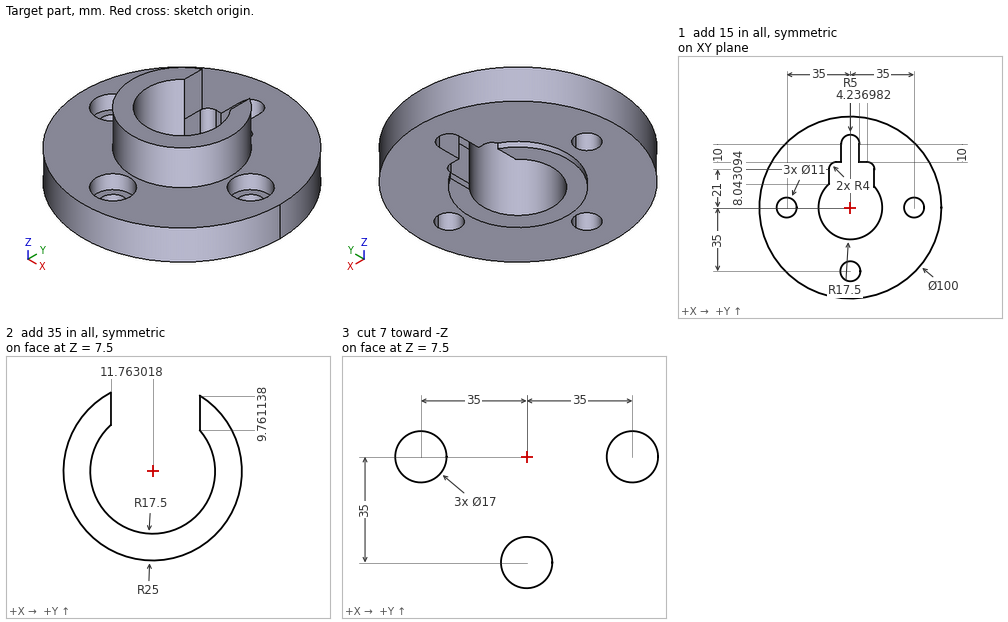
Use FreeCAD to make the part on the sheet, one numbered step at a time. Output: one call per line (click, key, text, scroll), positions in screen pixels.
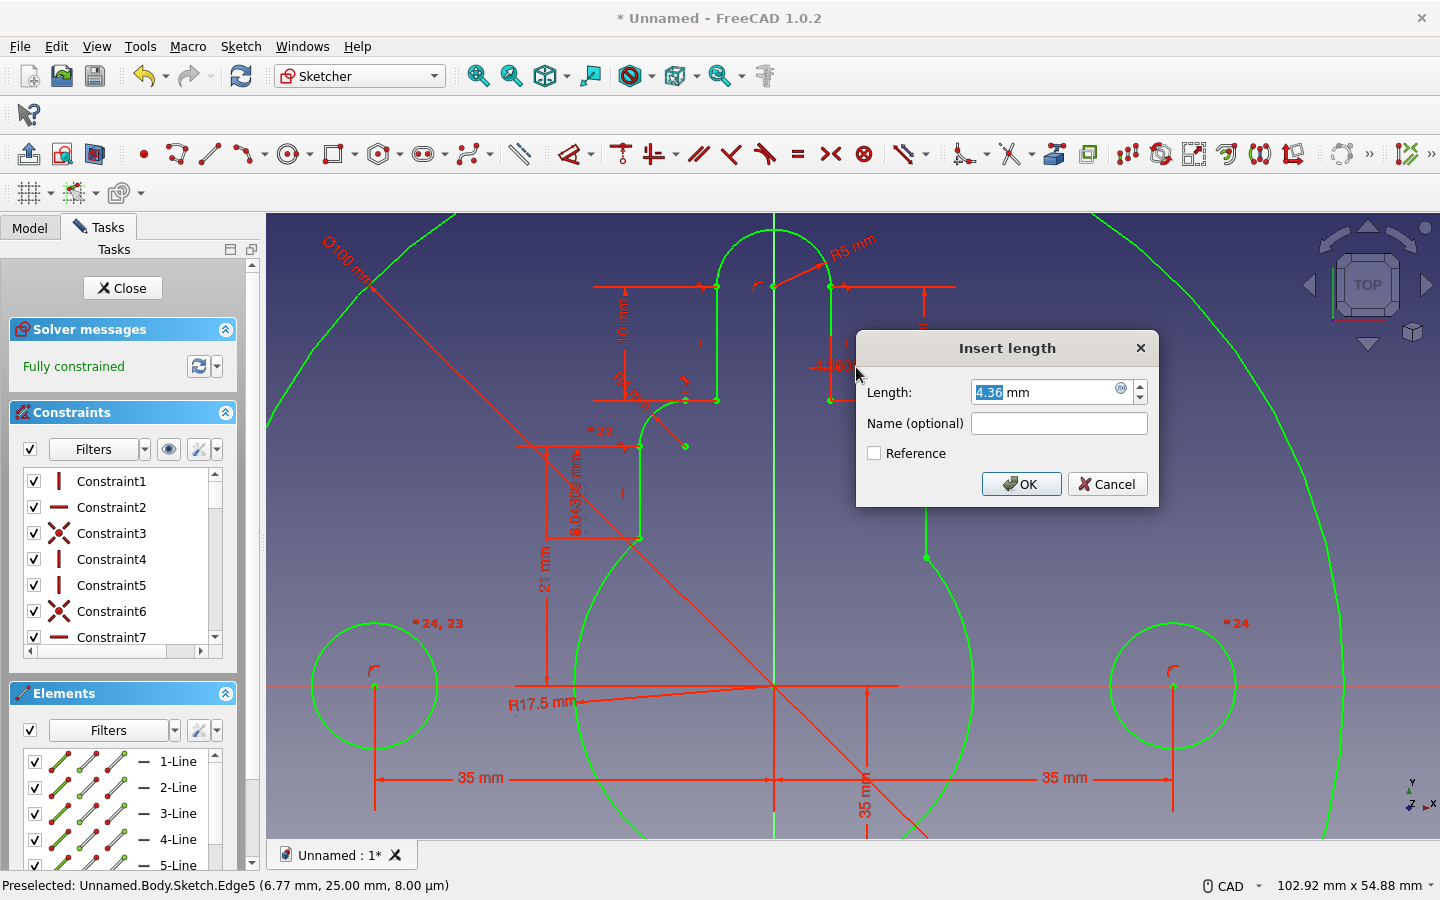
text(4.236982)
key(Return)
key(Escape)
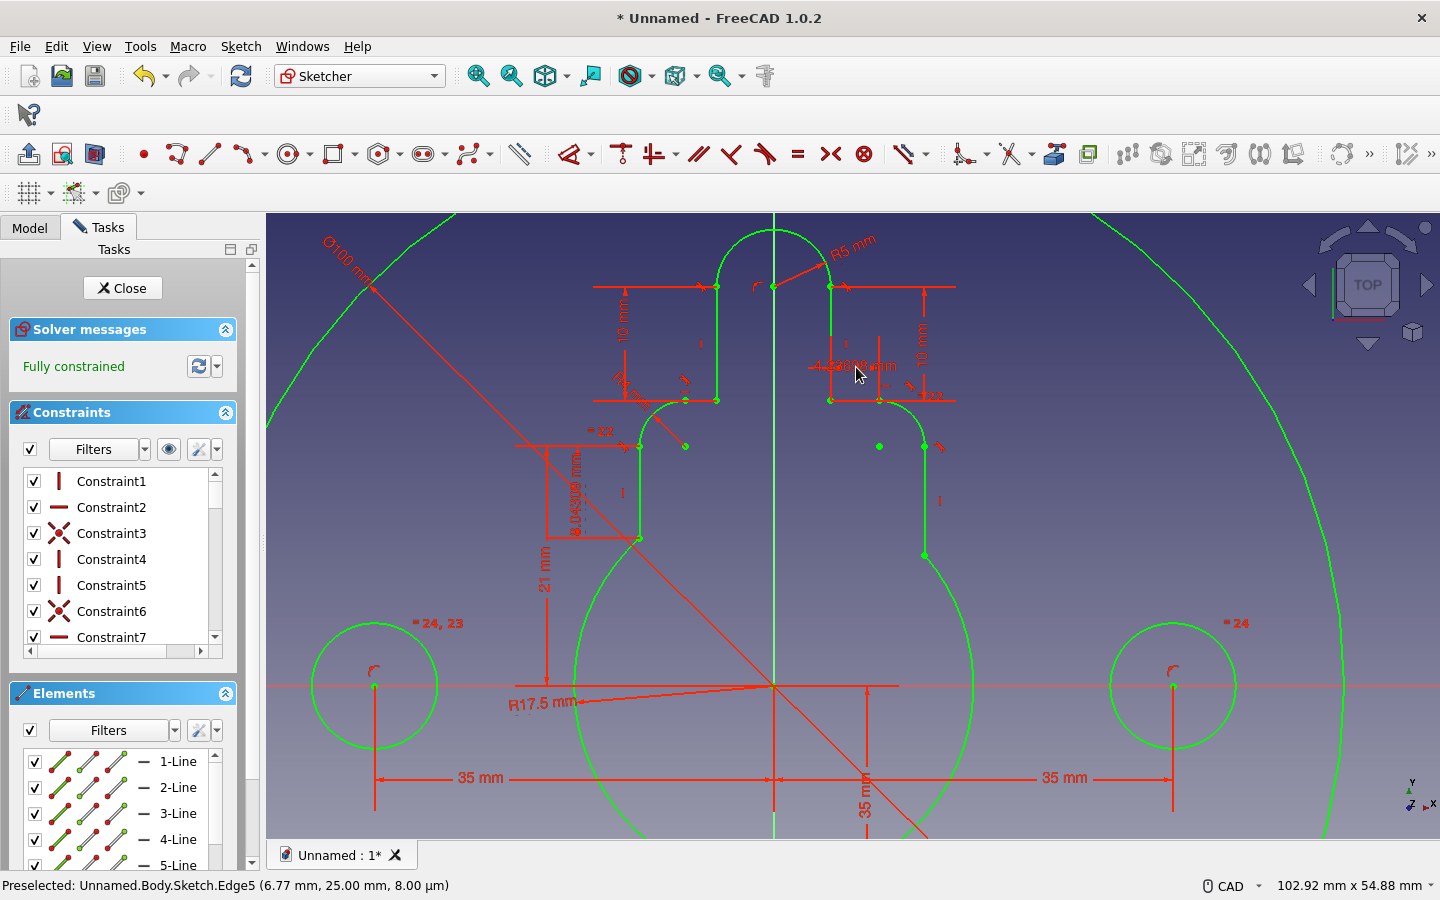
click(123, 288)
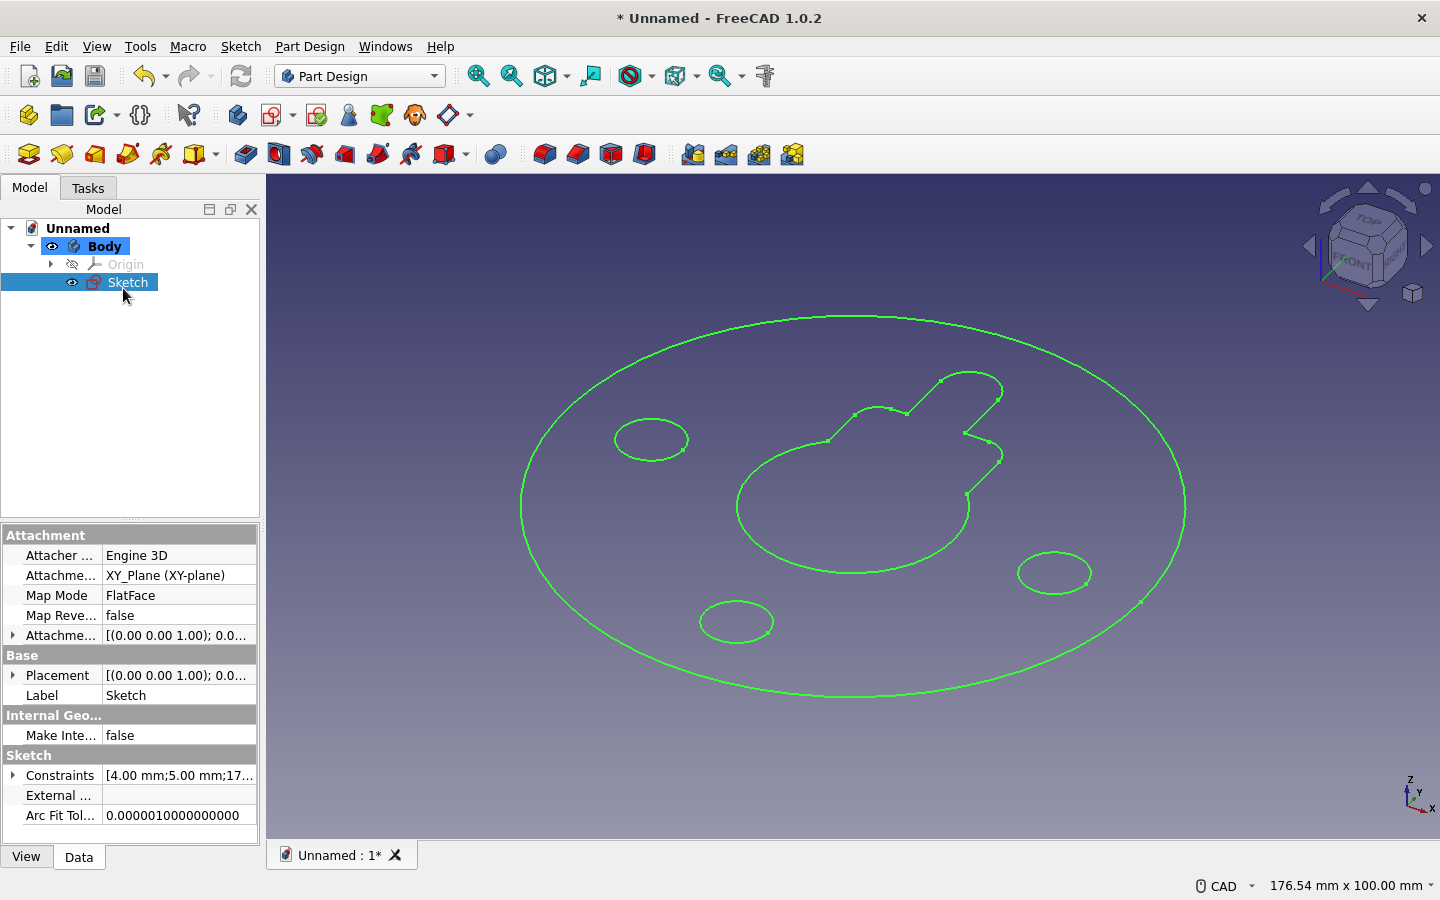
click(29, 154)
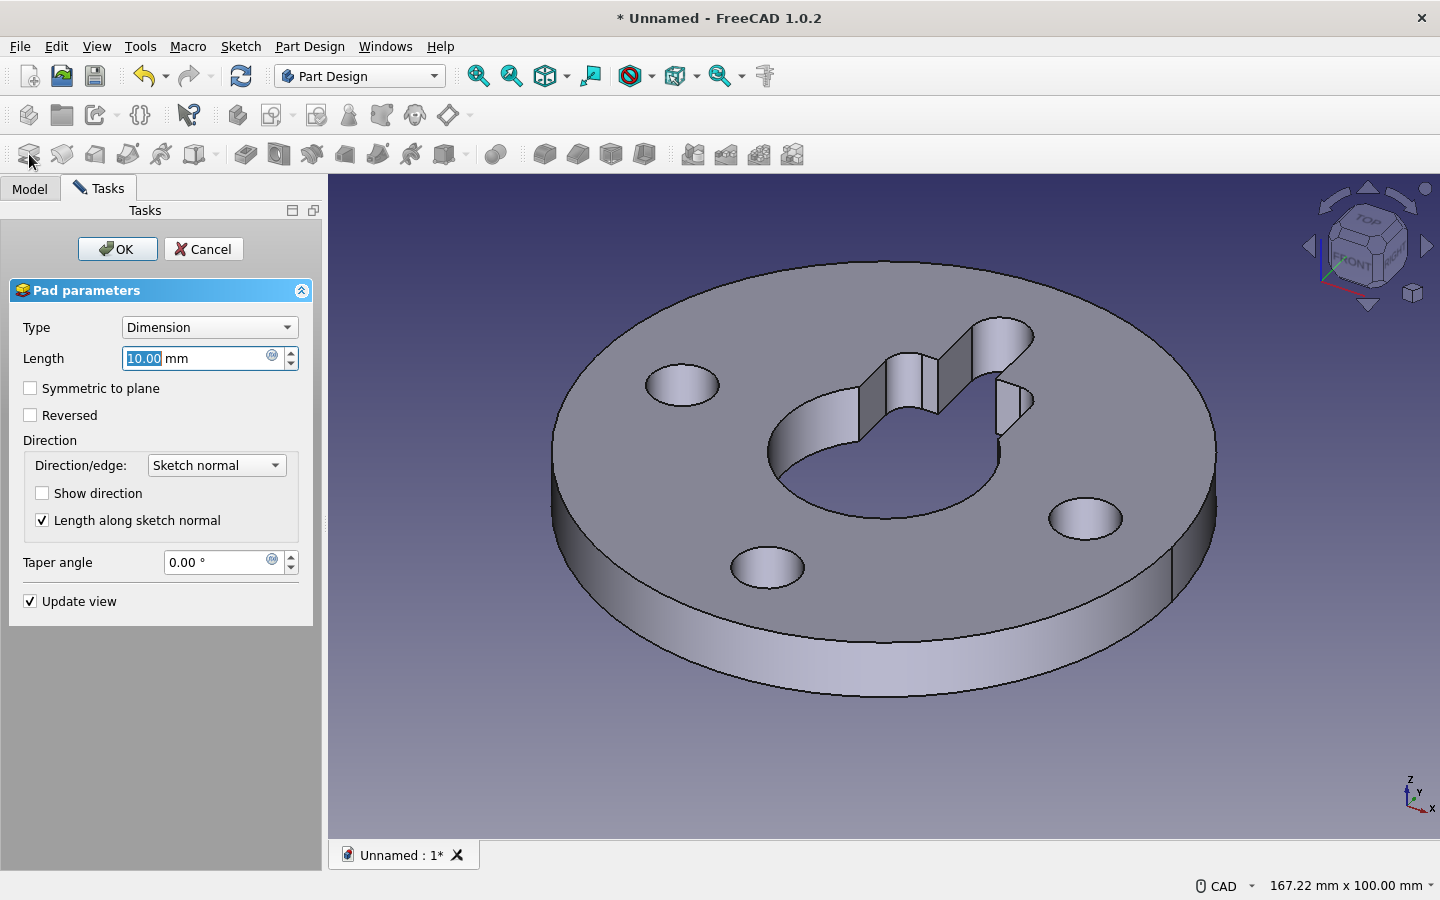
text(15)
key(Tab)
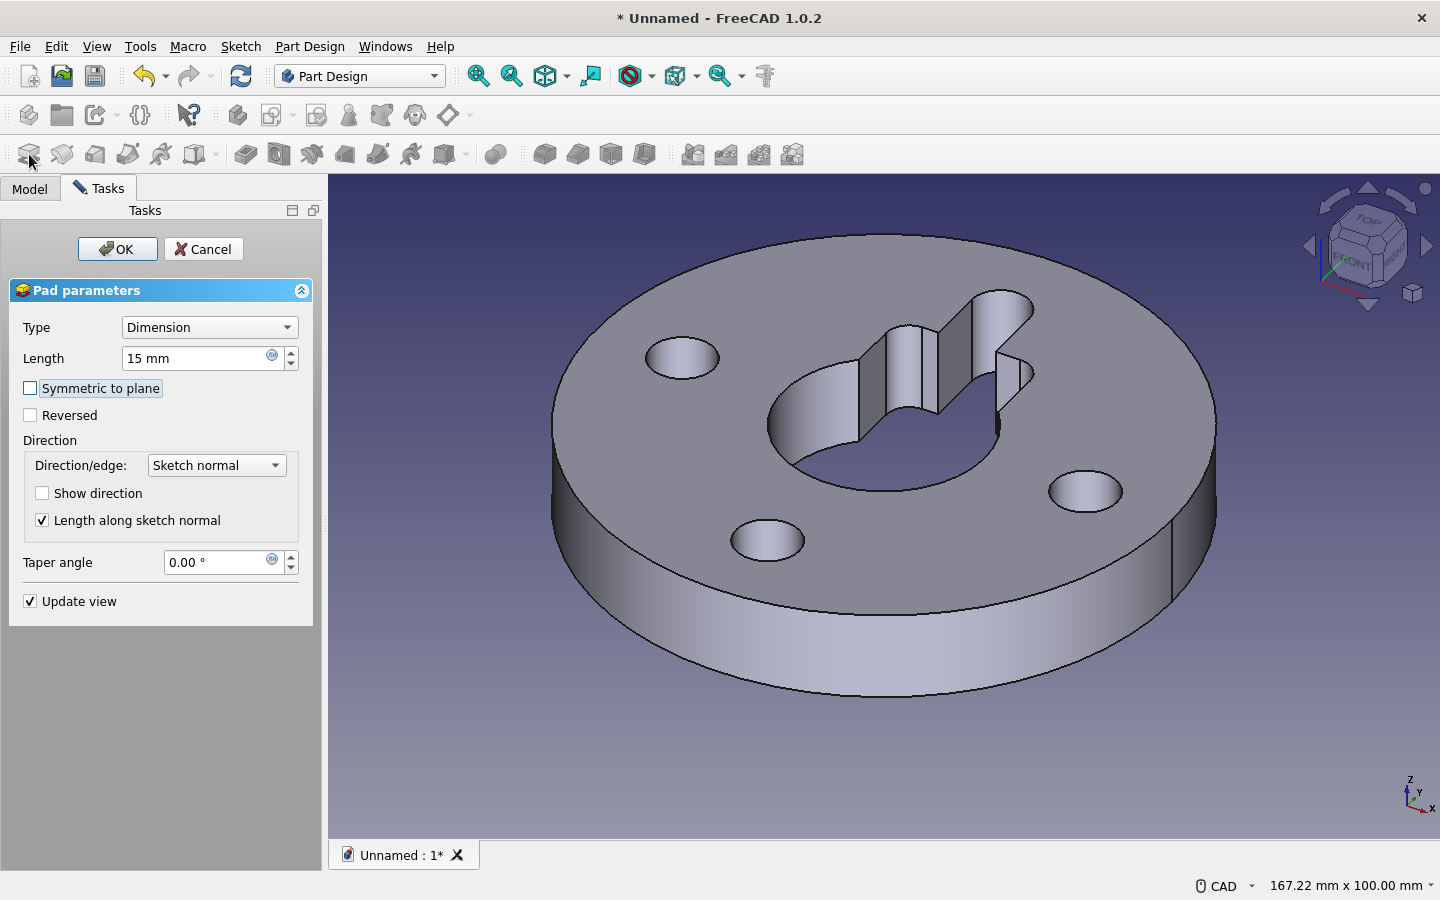
click(31, 388)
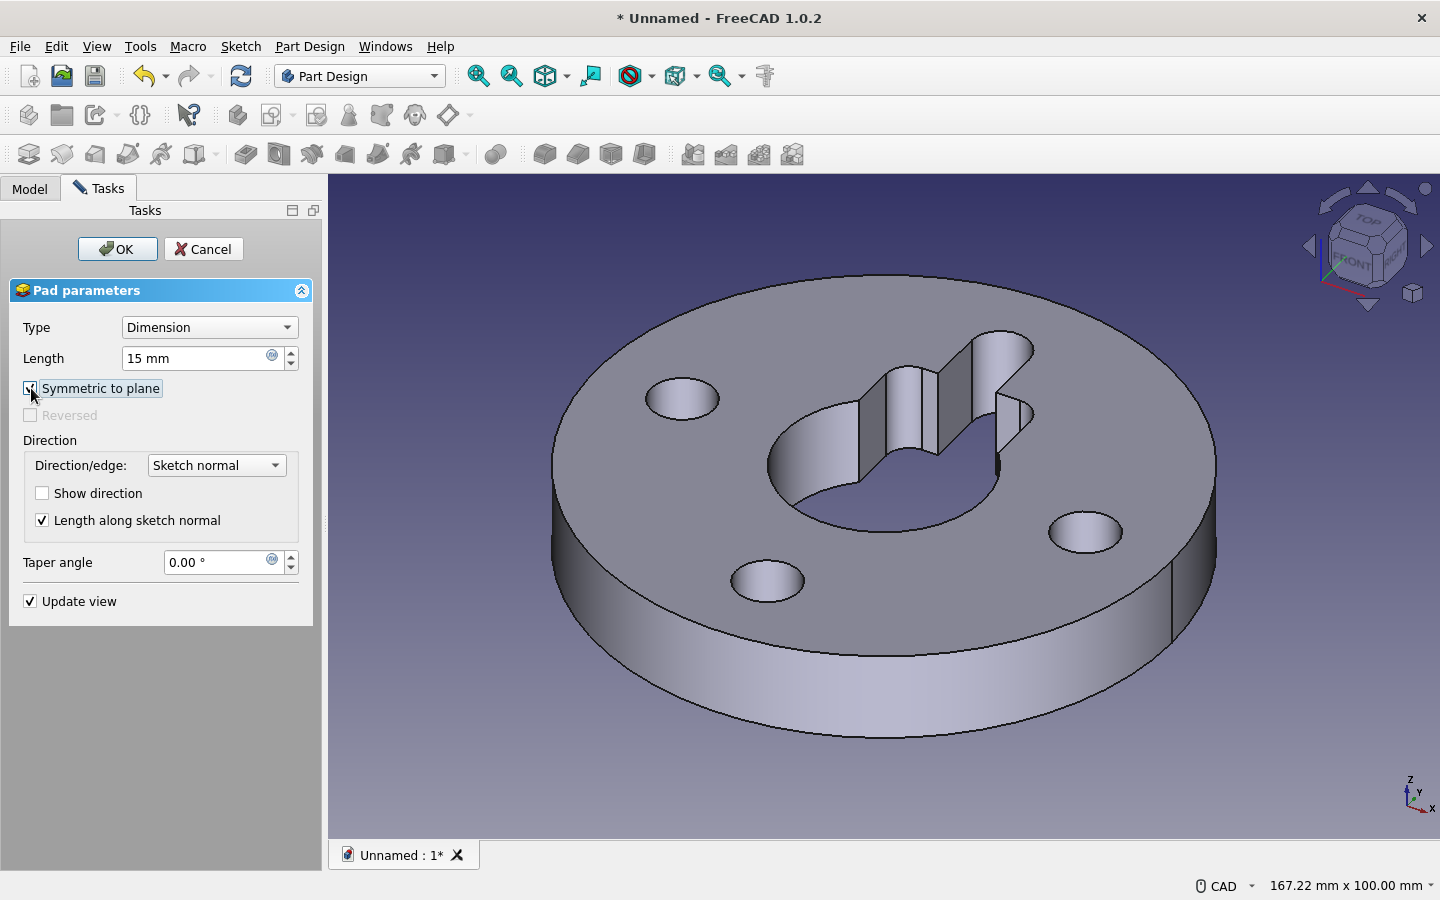
click(118, 249)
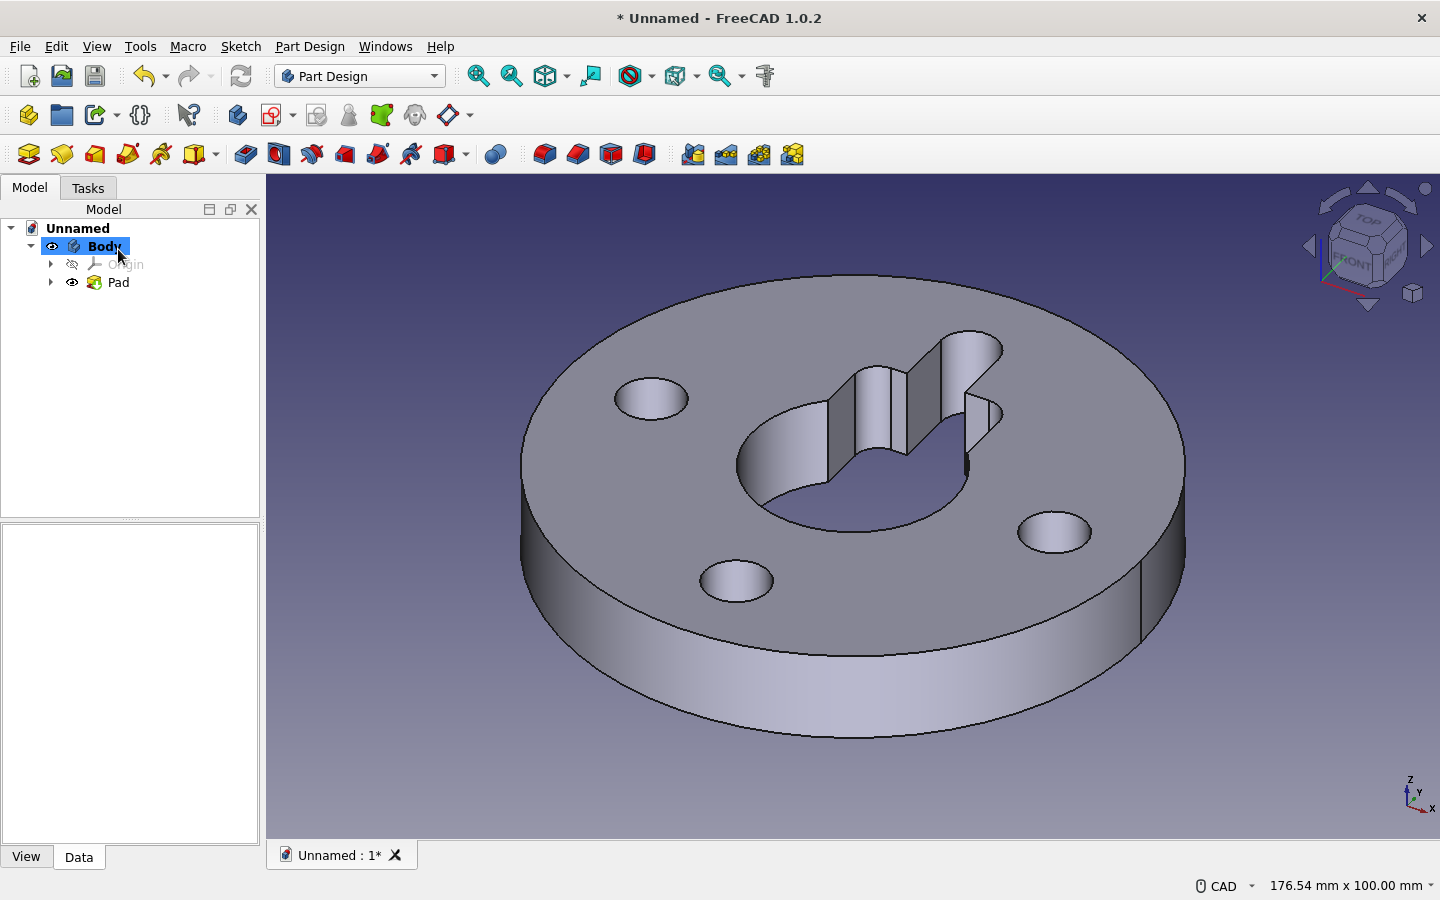
click(1065, 472)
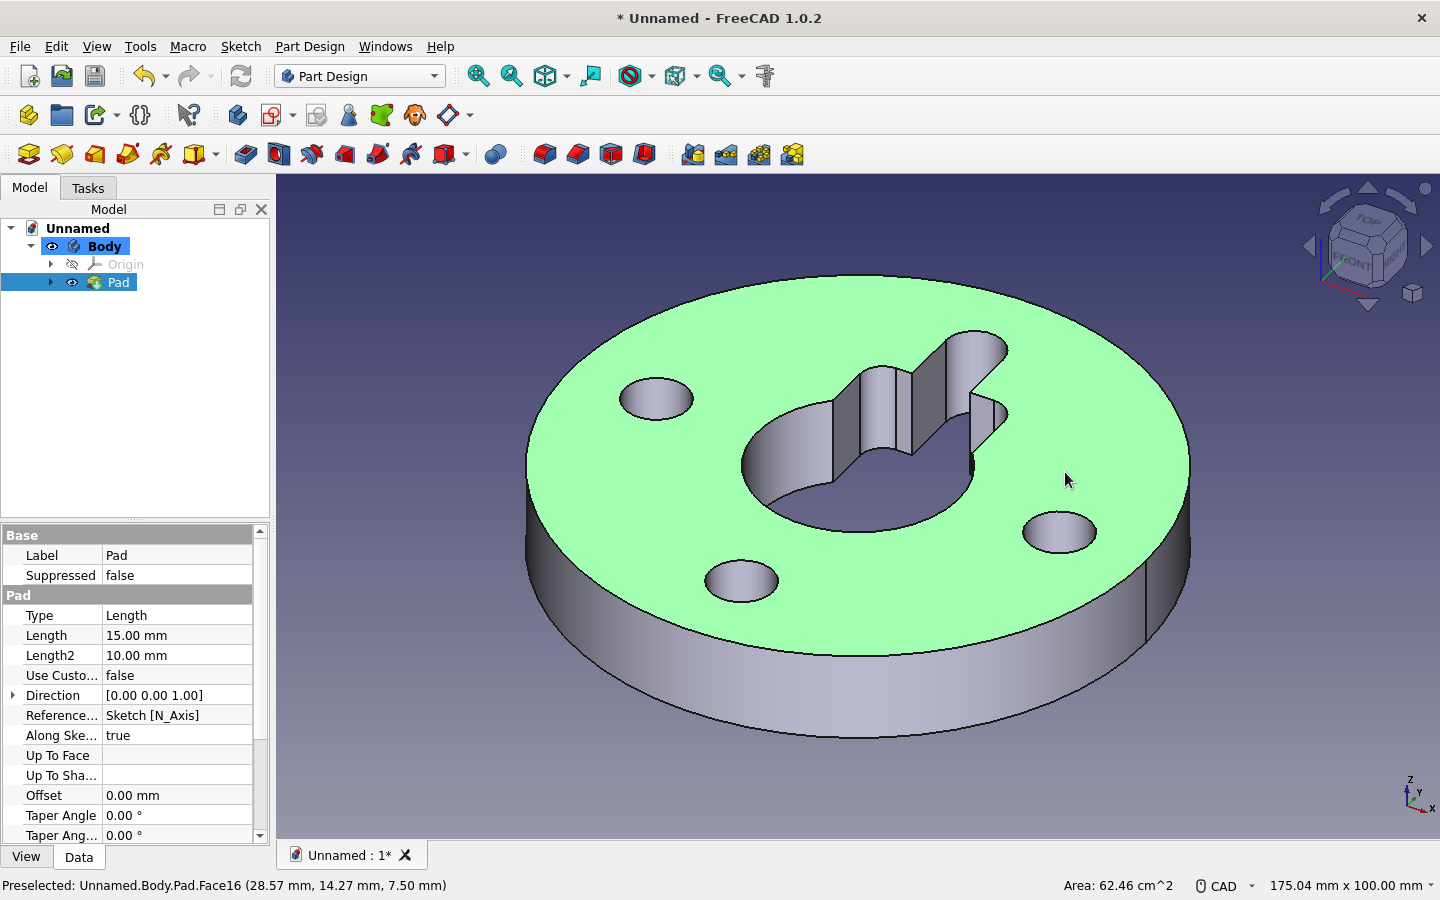
click(270, 116)